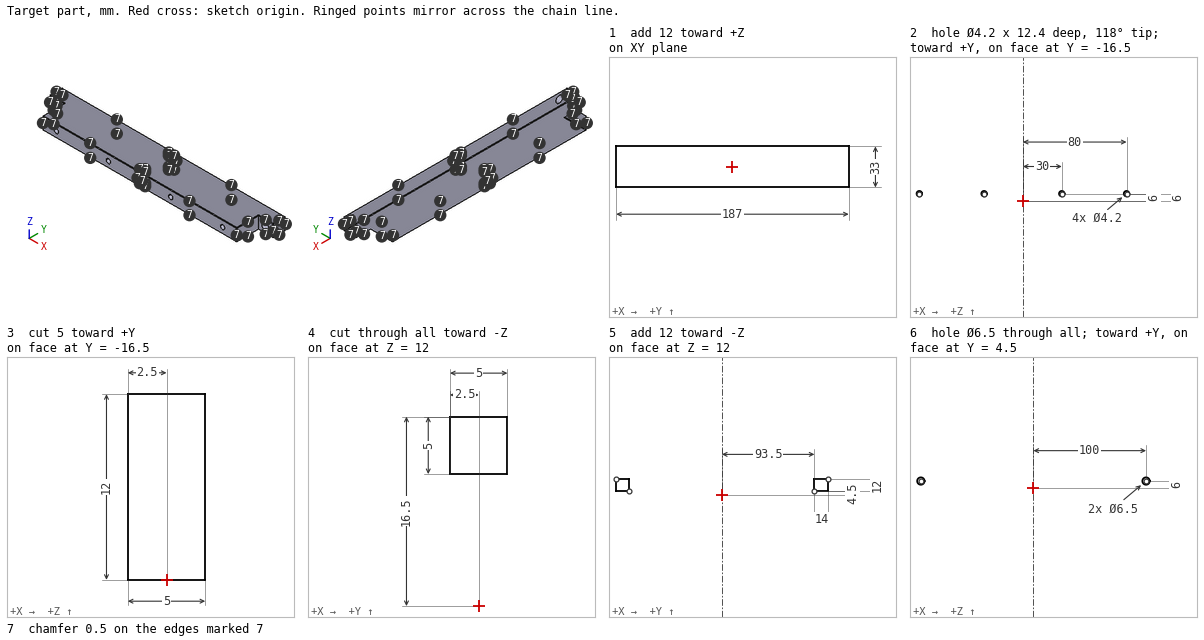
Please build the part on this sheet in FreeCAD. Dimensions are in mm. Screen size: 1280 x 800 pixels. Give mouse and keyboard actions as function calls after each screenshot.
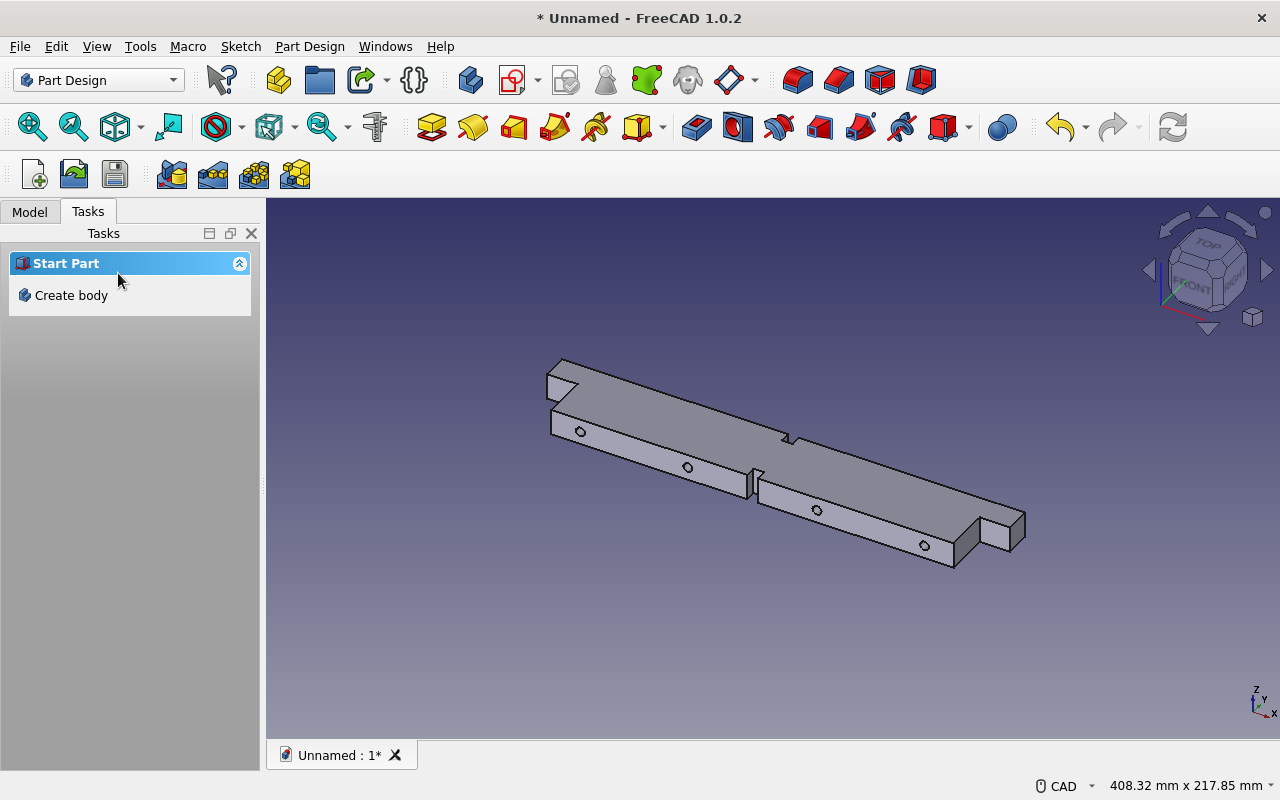
click(995, 534)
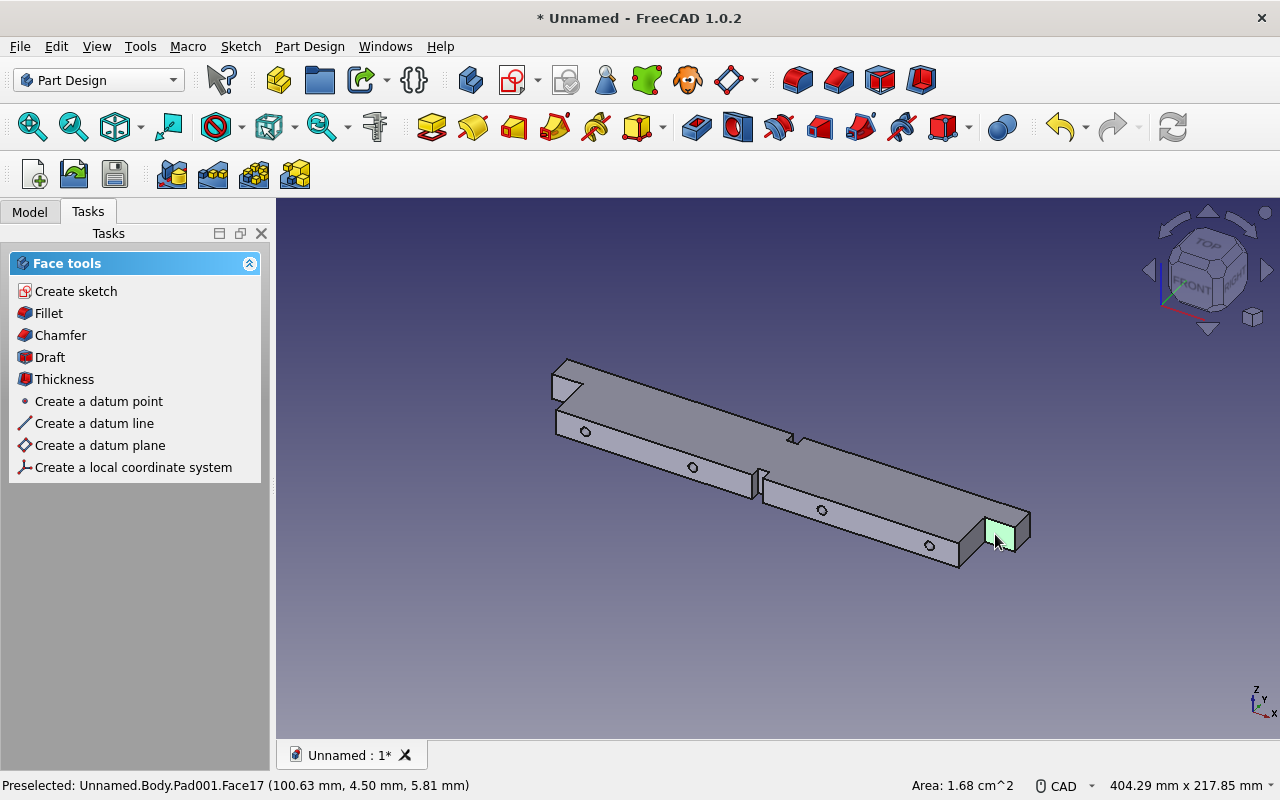
click(512, 80)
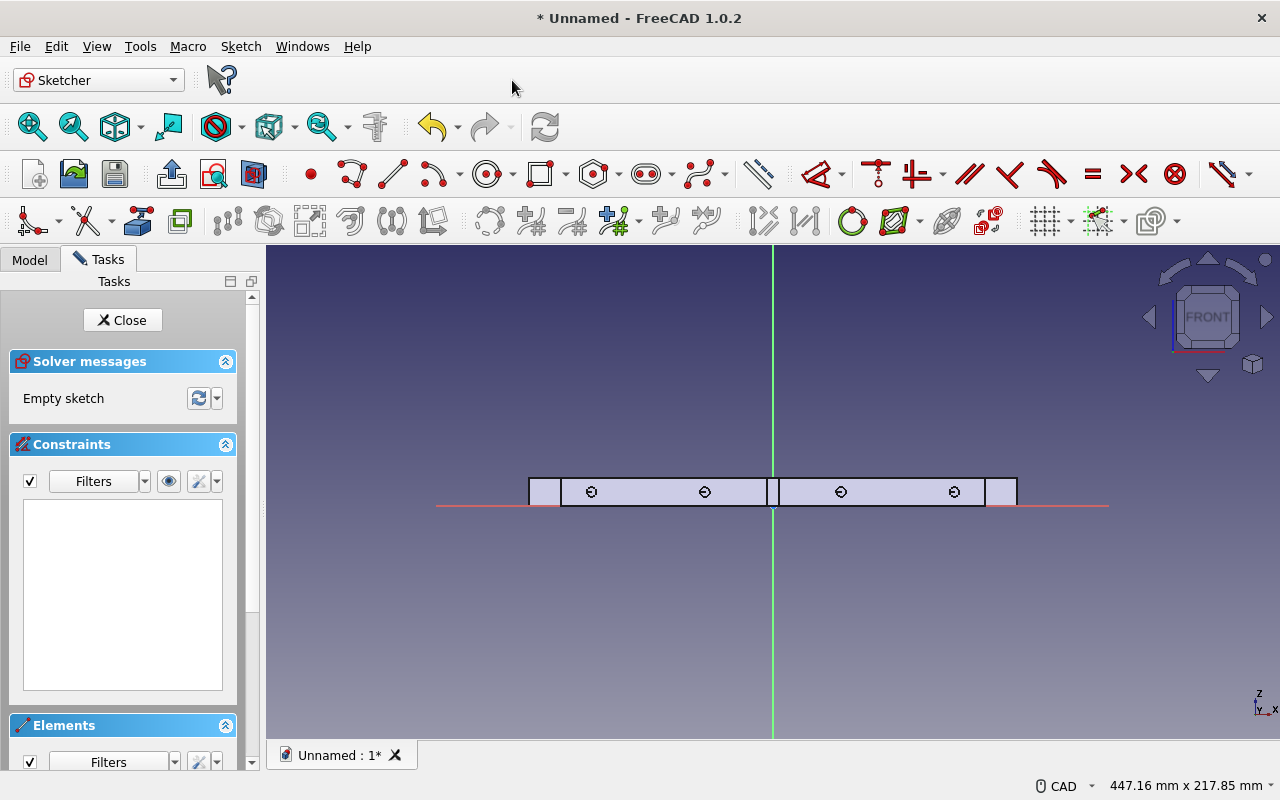
key(g)
key(c)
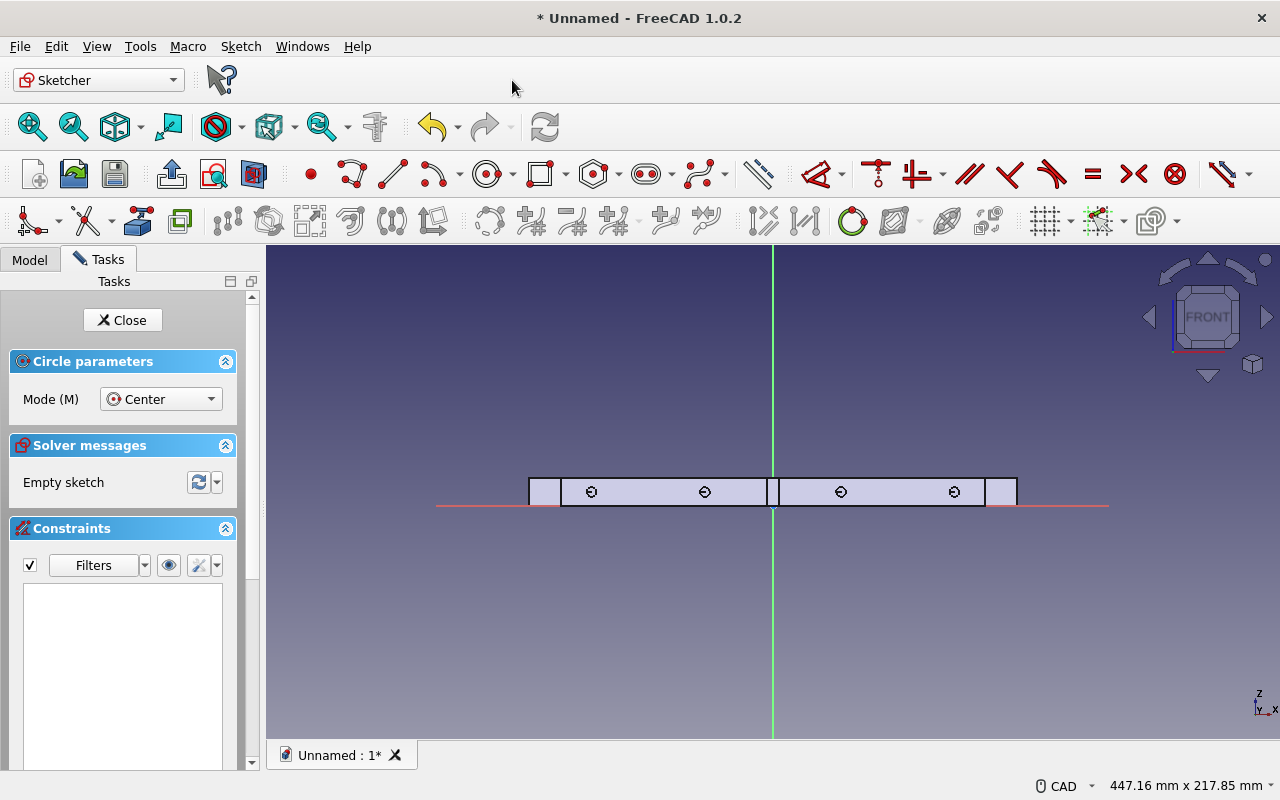
scroll(1000, 492, up, 6)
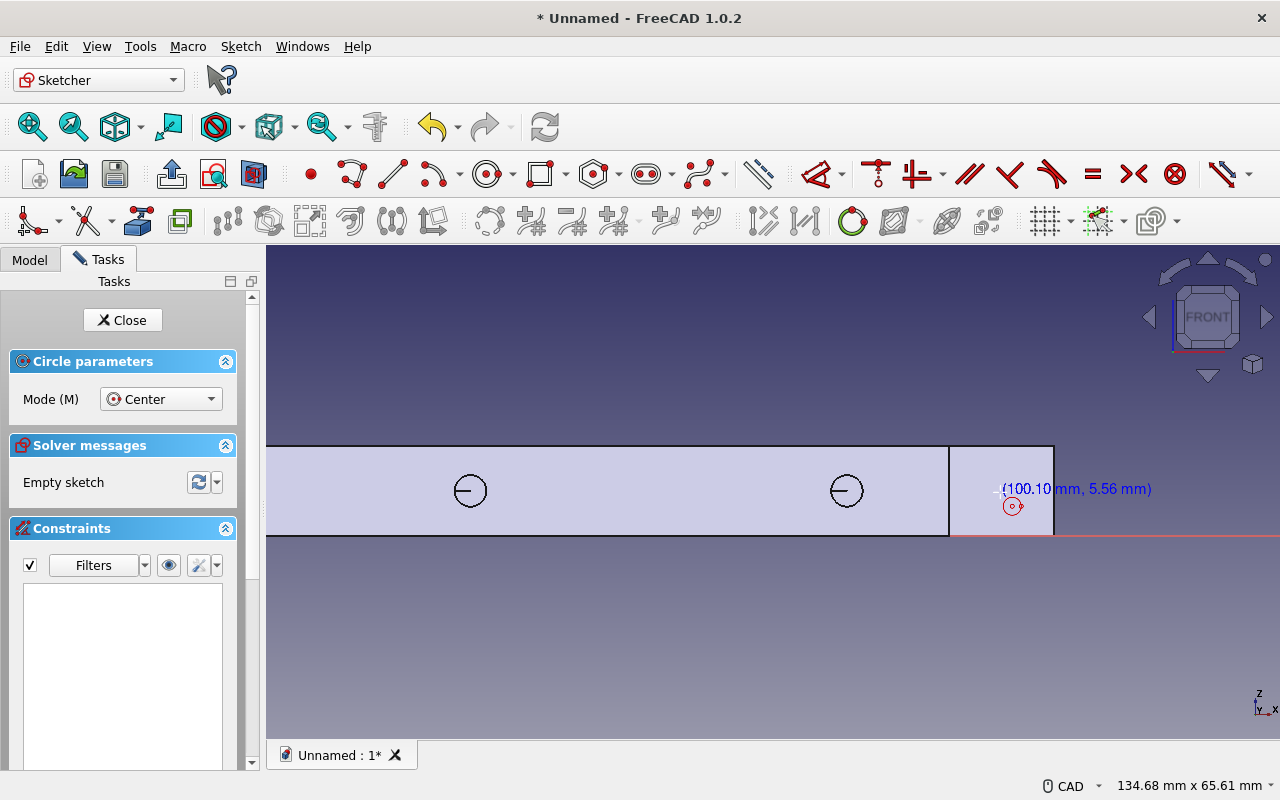
click(998, 491)
click(1015, 474)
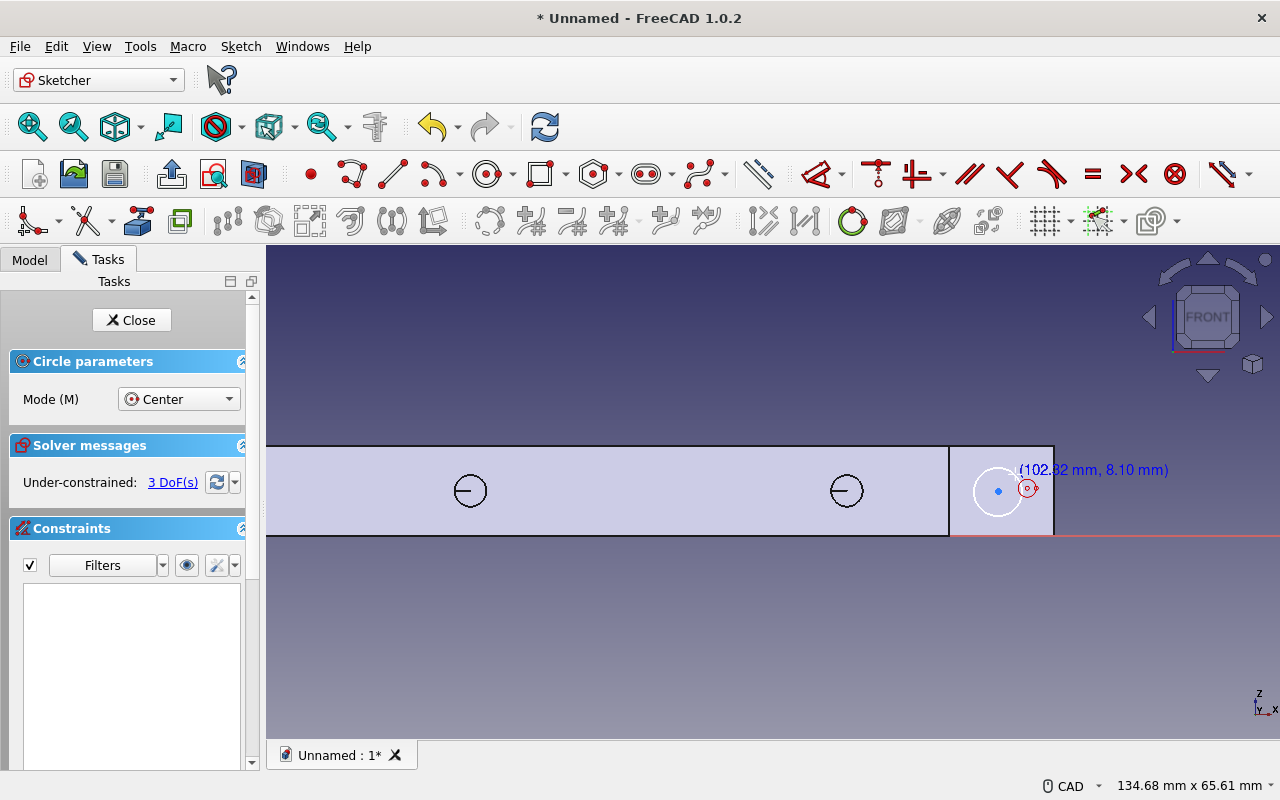
scroll(972, 487, down, 5)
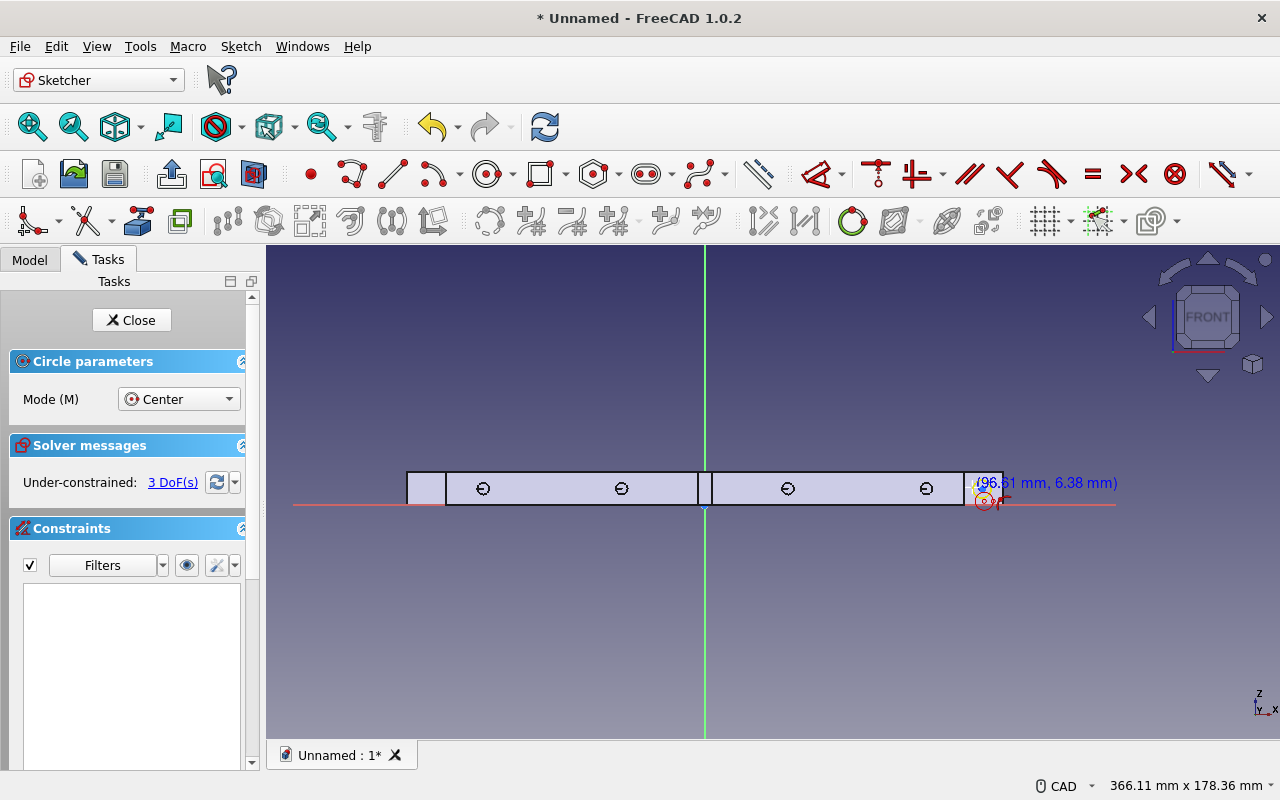
scroll(428, 489, up, 5)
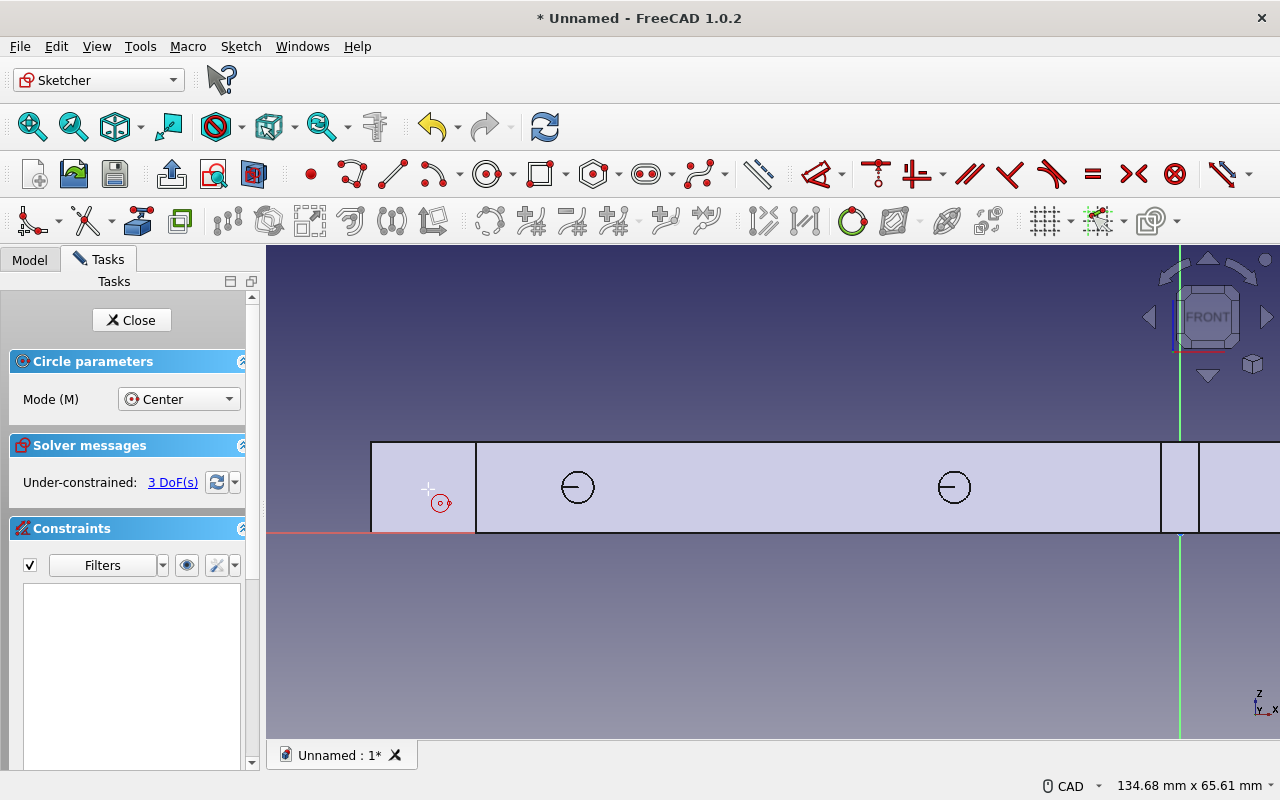
click(427, 487)
click(445, 470)
key(Escape)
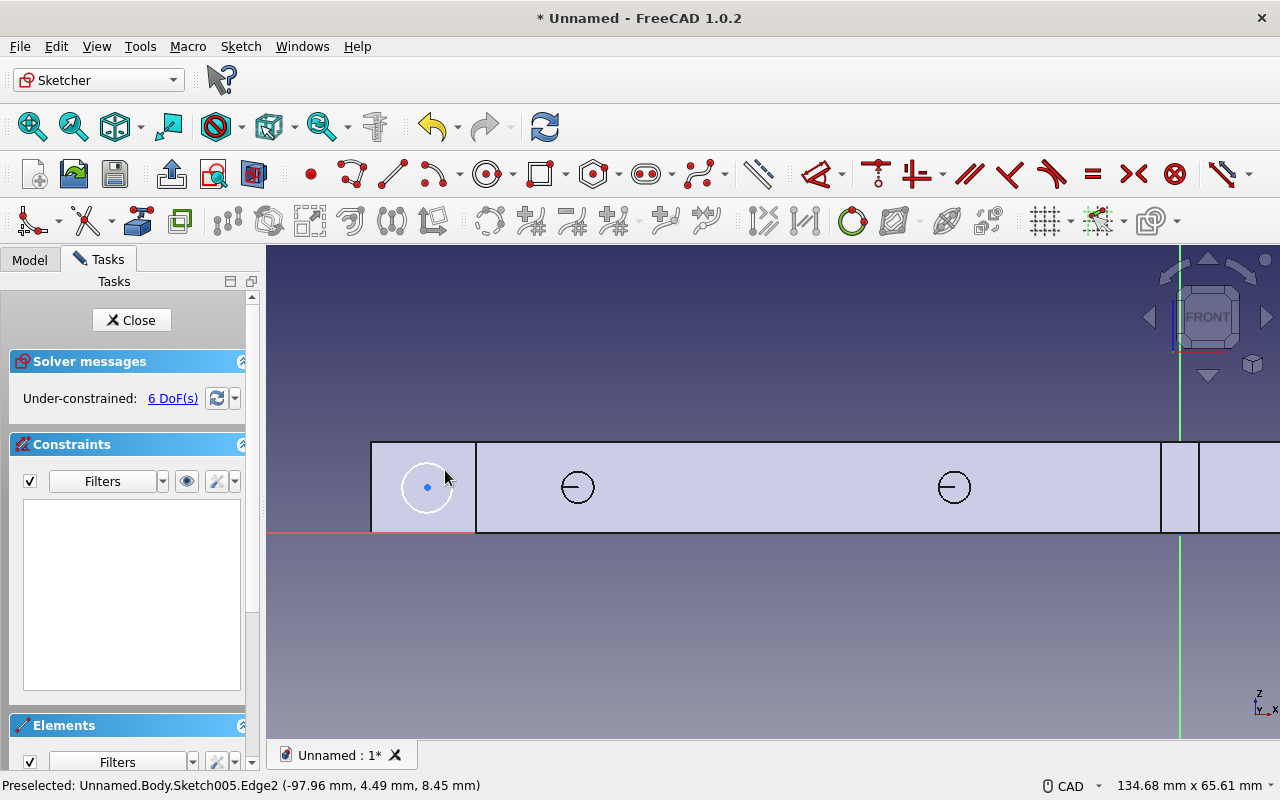
scroll(428, 489, down, 5)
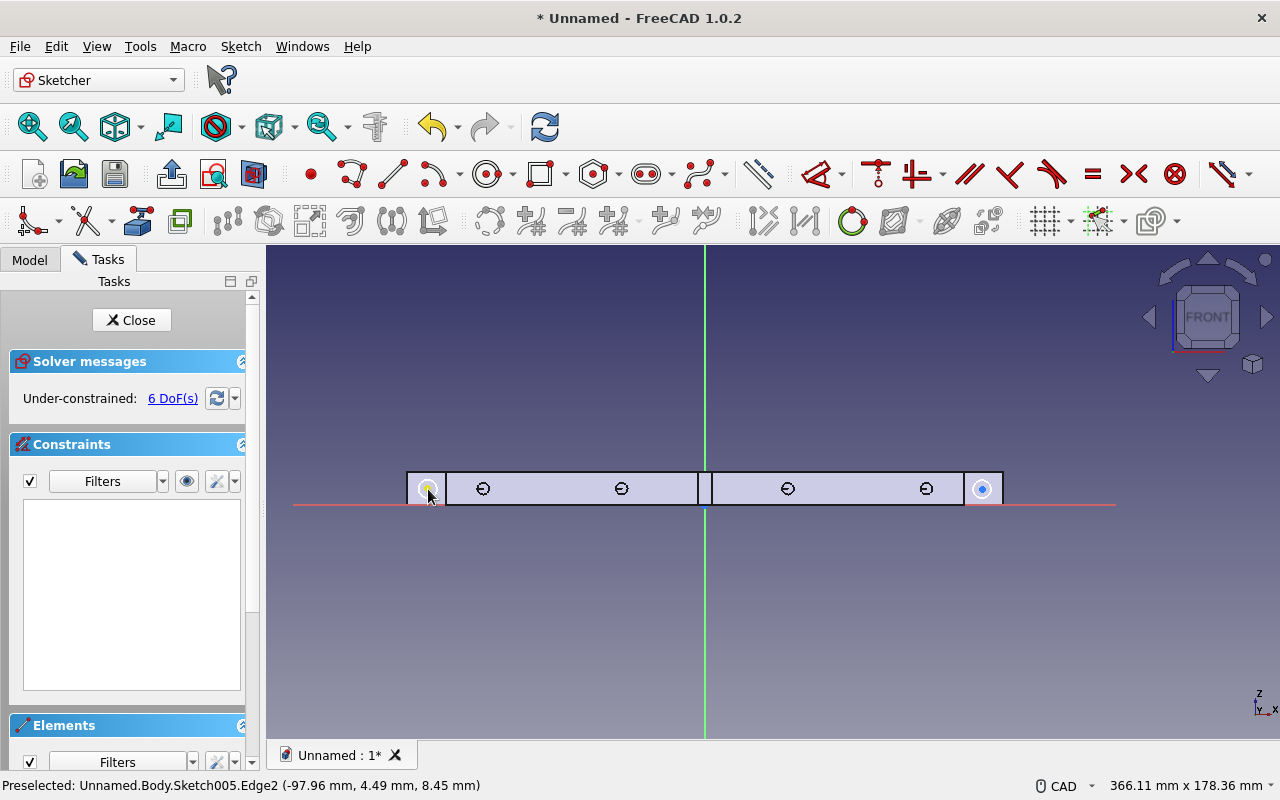
scroll(988, 483, up, 3)